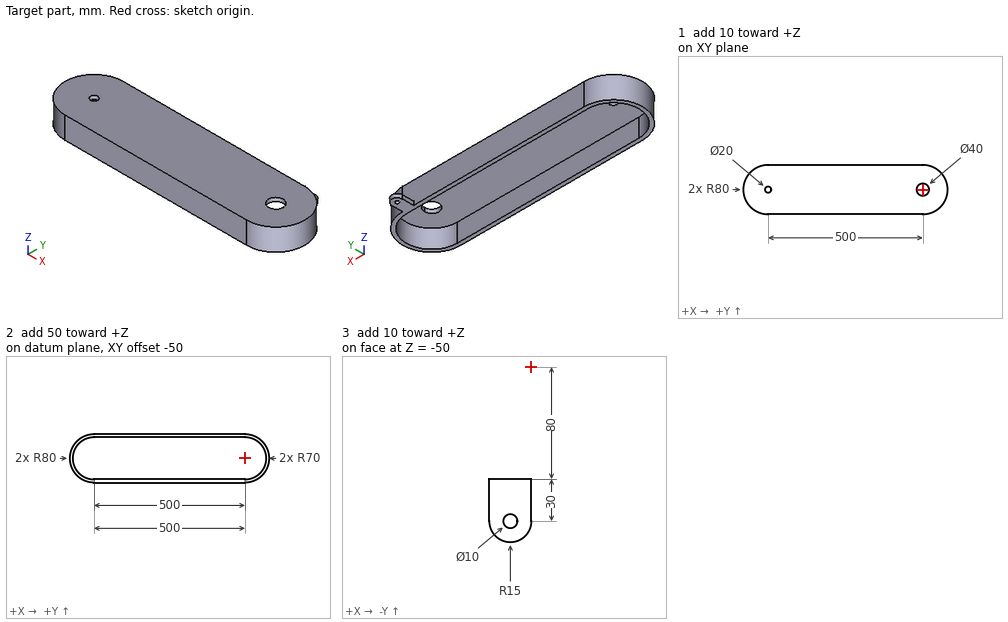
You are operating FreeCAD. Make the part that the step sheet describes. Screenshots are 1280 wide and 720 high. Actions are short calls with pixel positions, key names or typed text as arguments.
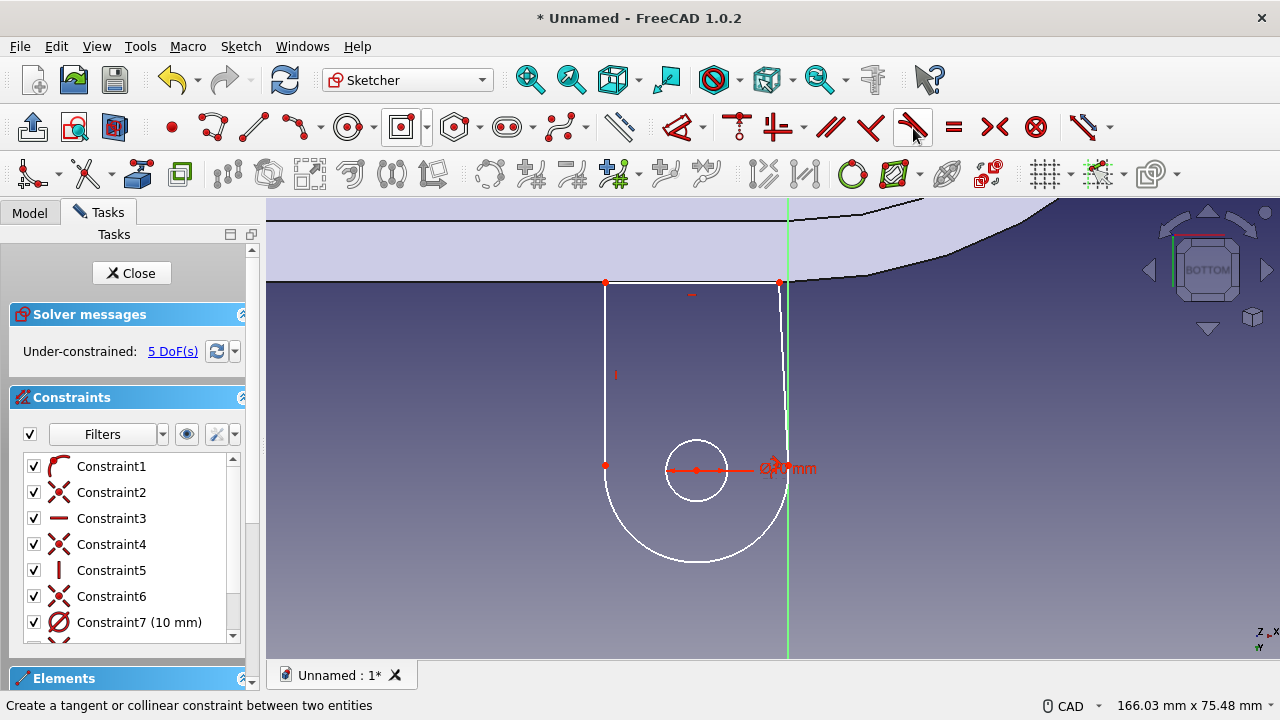
click(605, 338)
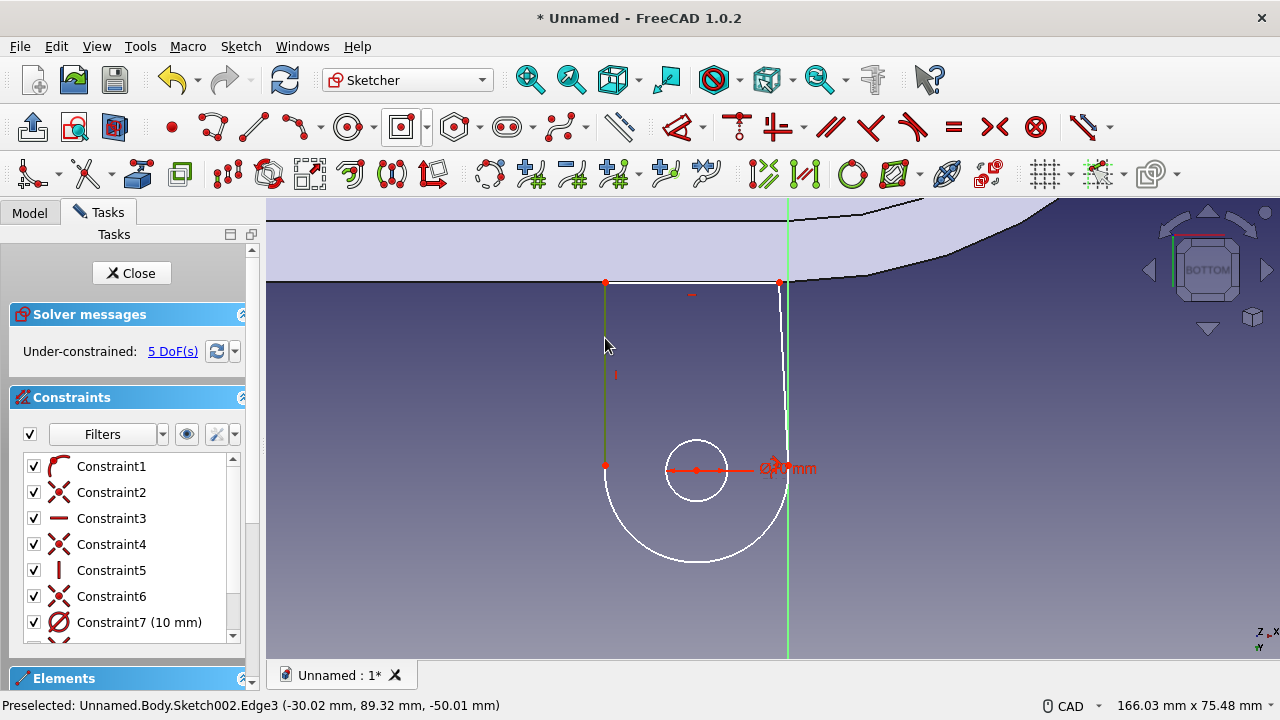
click(641, 544)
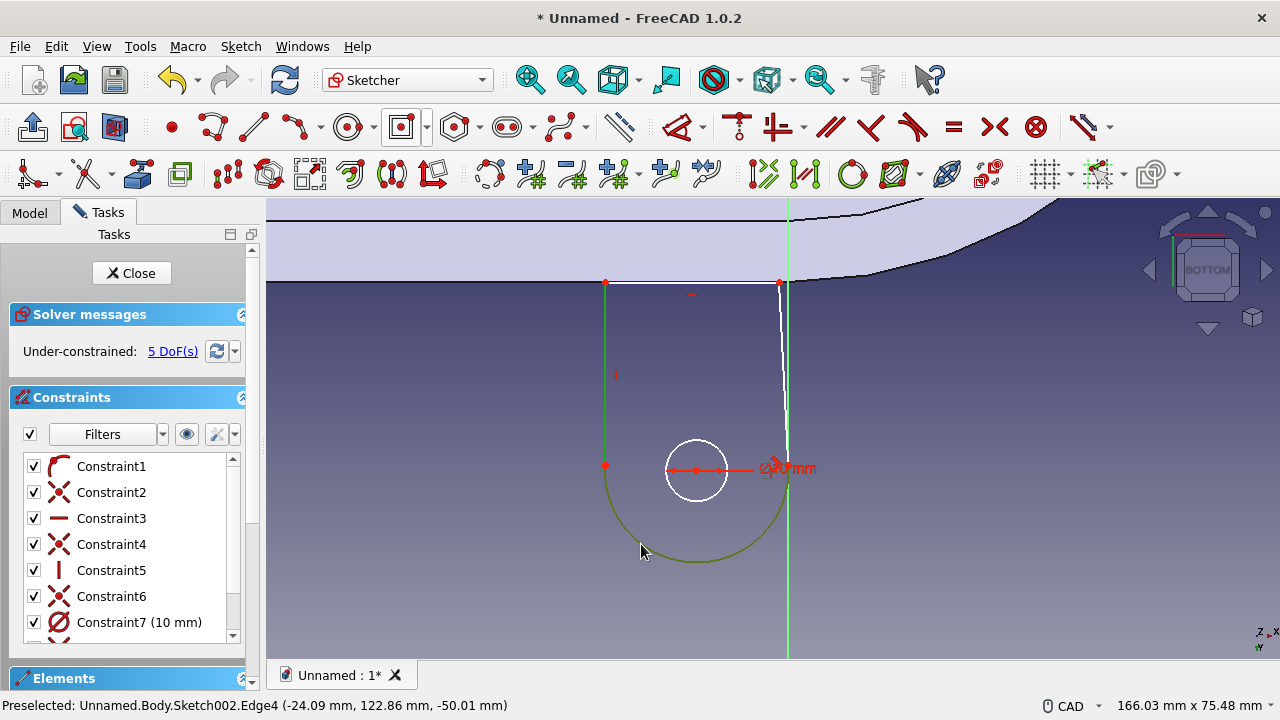
key(t)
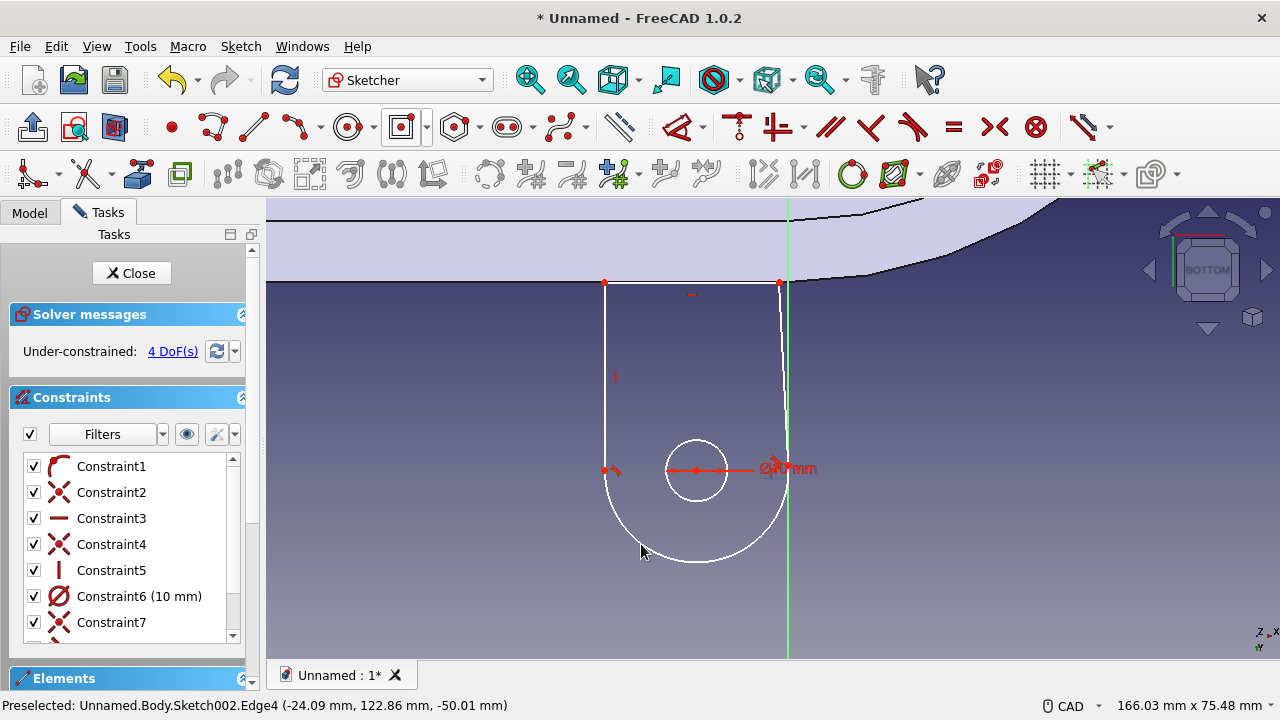
click(786, 411)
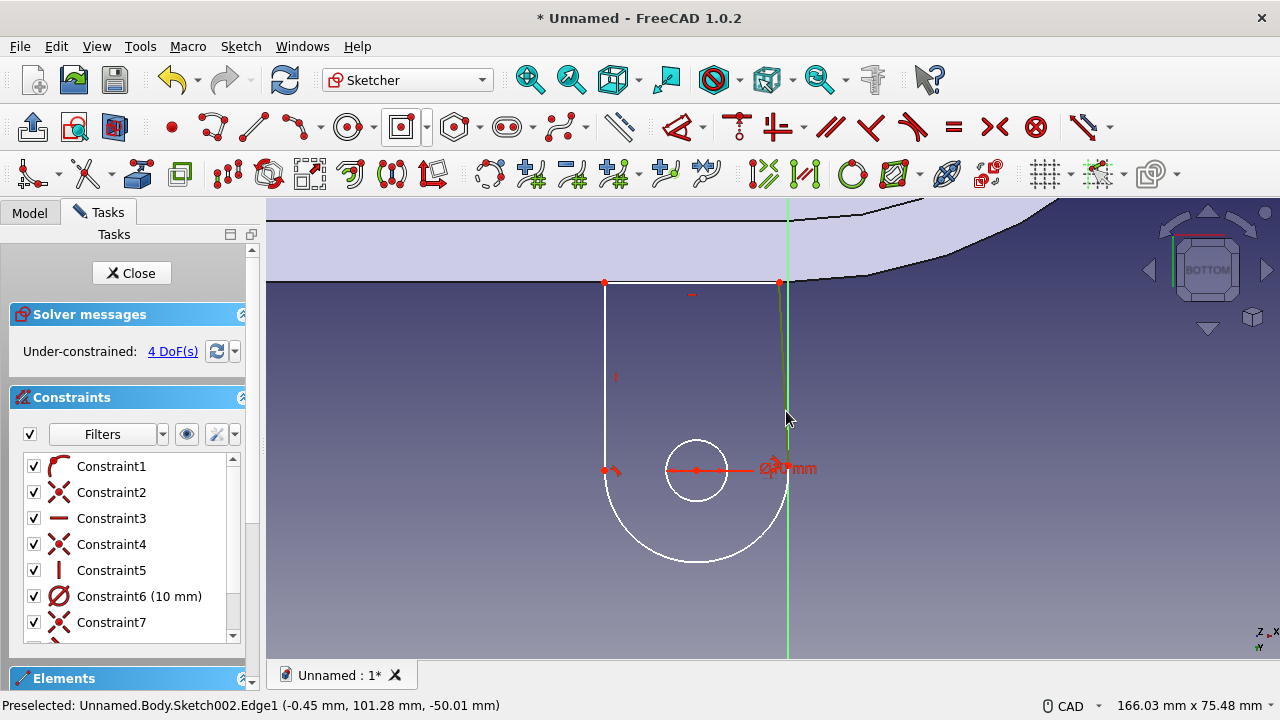
key(v)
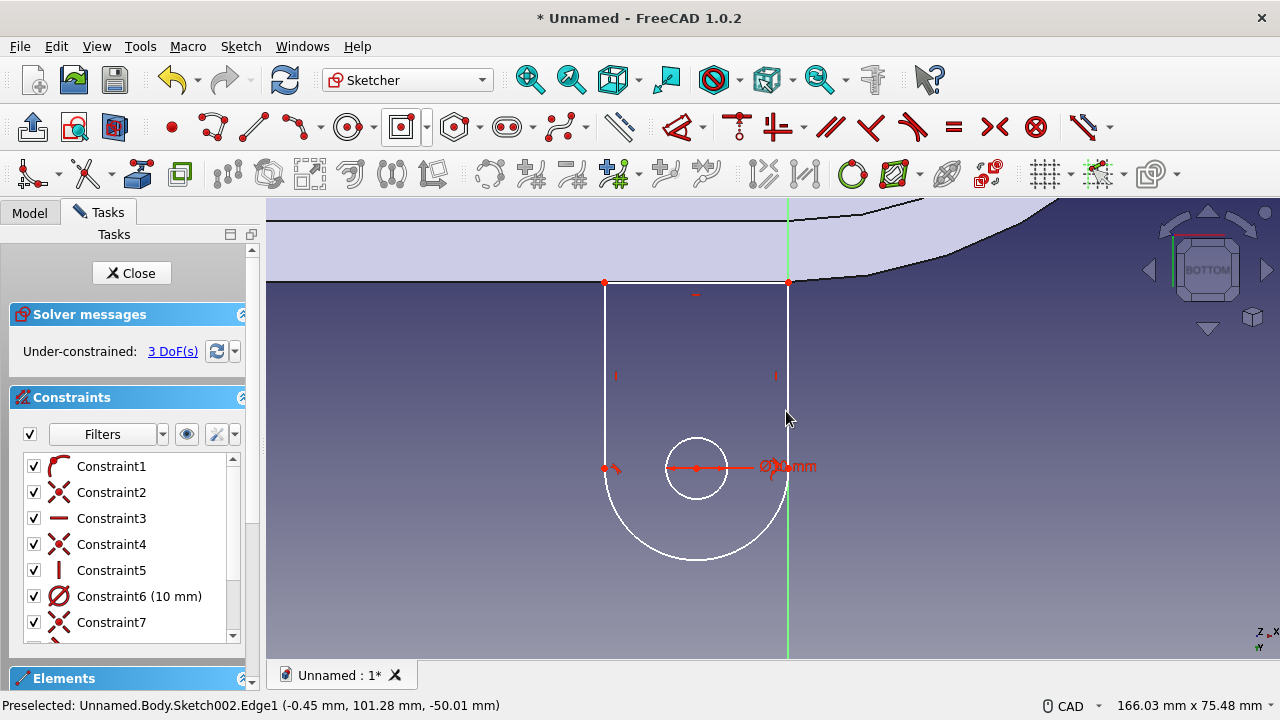
click(676, 128)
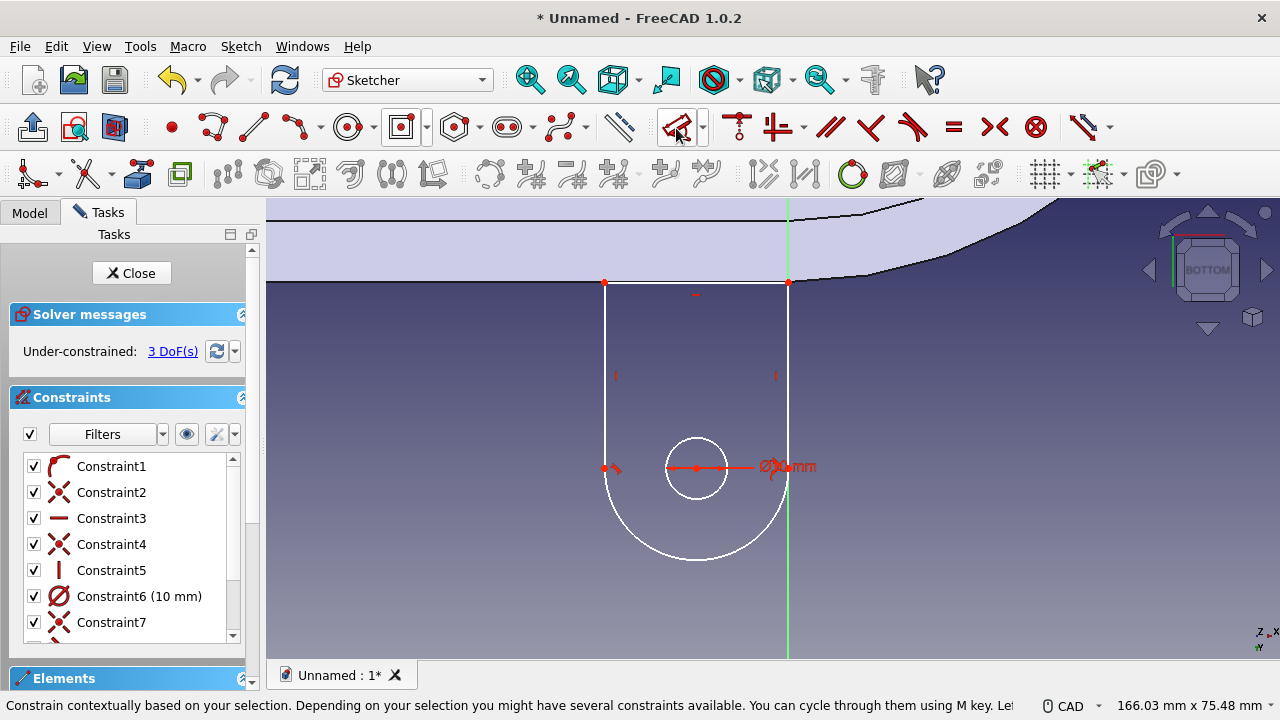
click(643, 543)
click(624, 569)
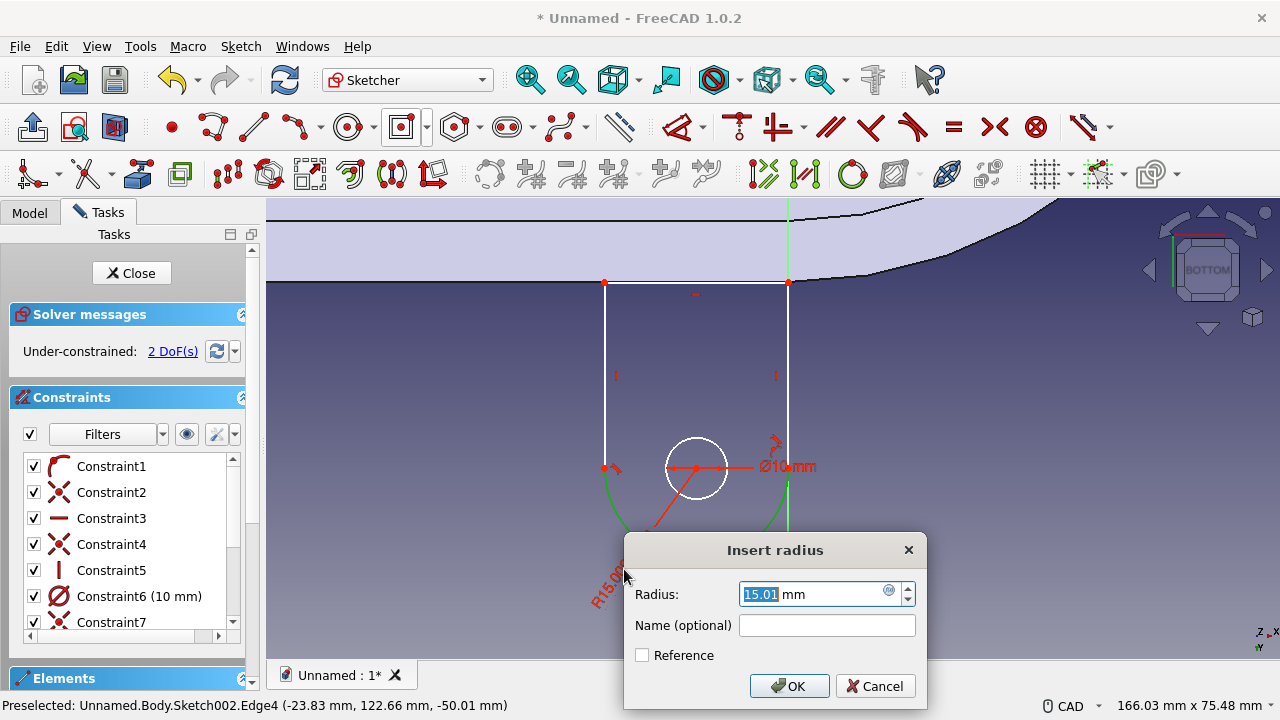
text(15)
key(Return)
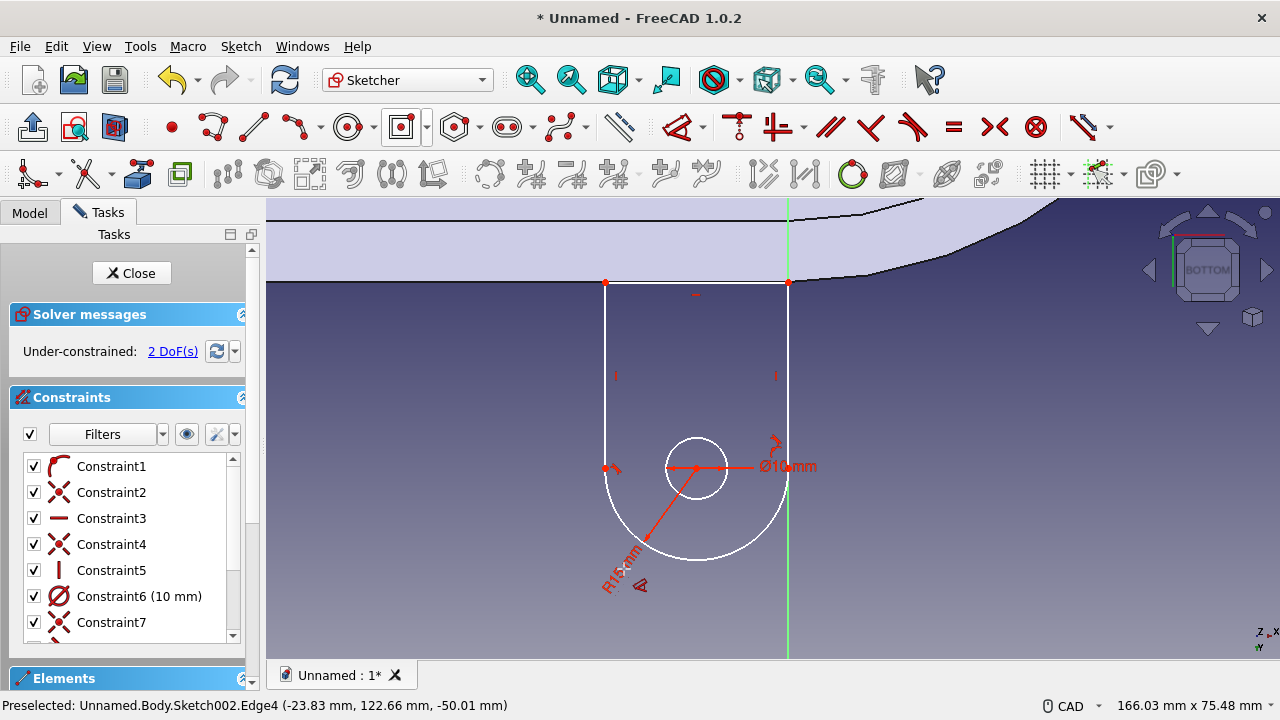
click(788, 413)
click(822, 376)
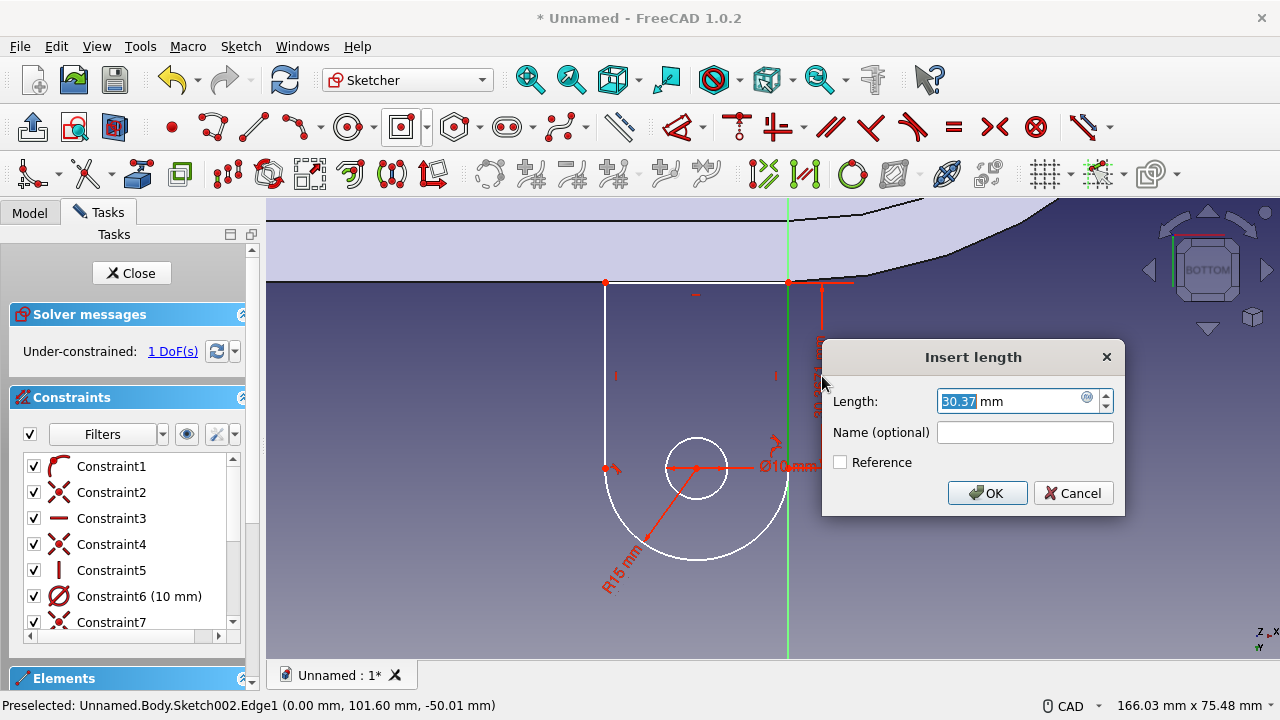
text(30)
key(Return)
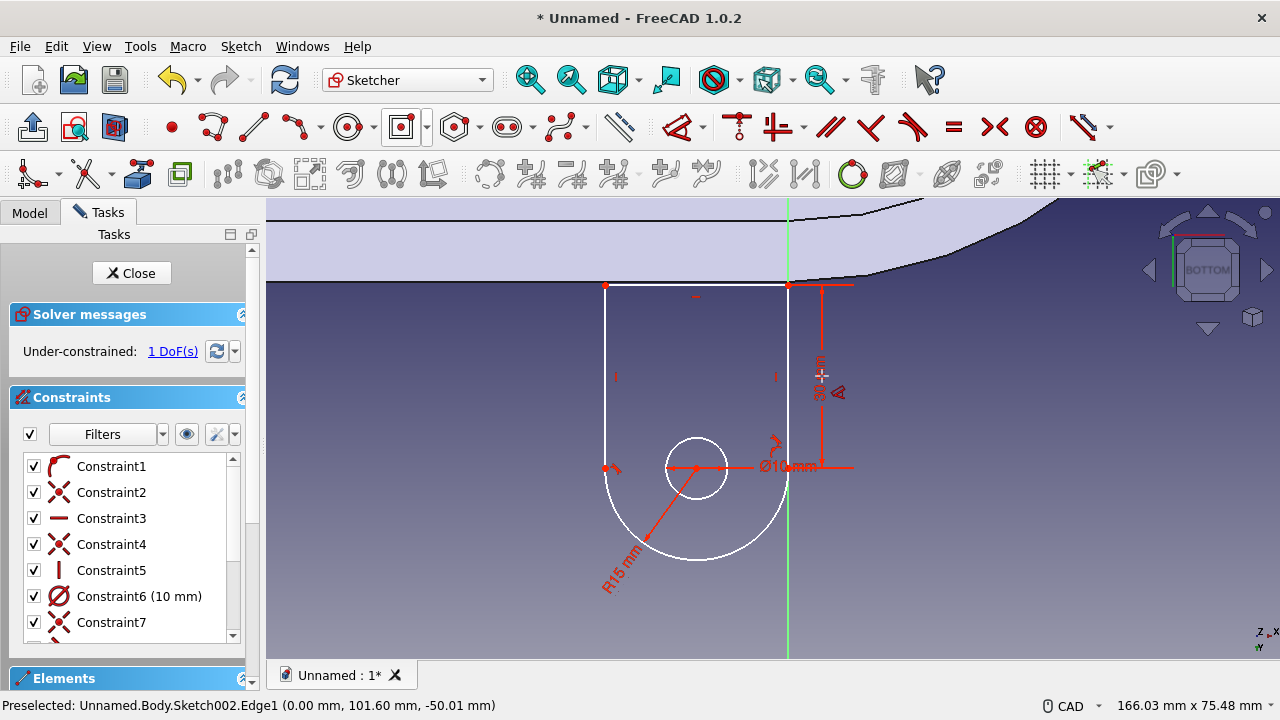
click(788, 285)
click(822, 256)